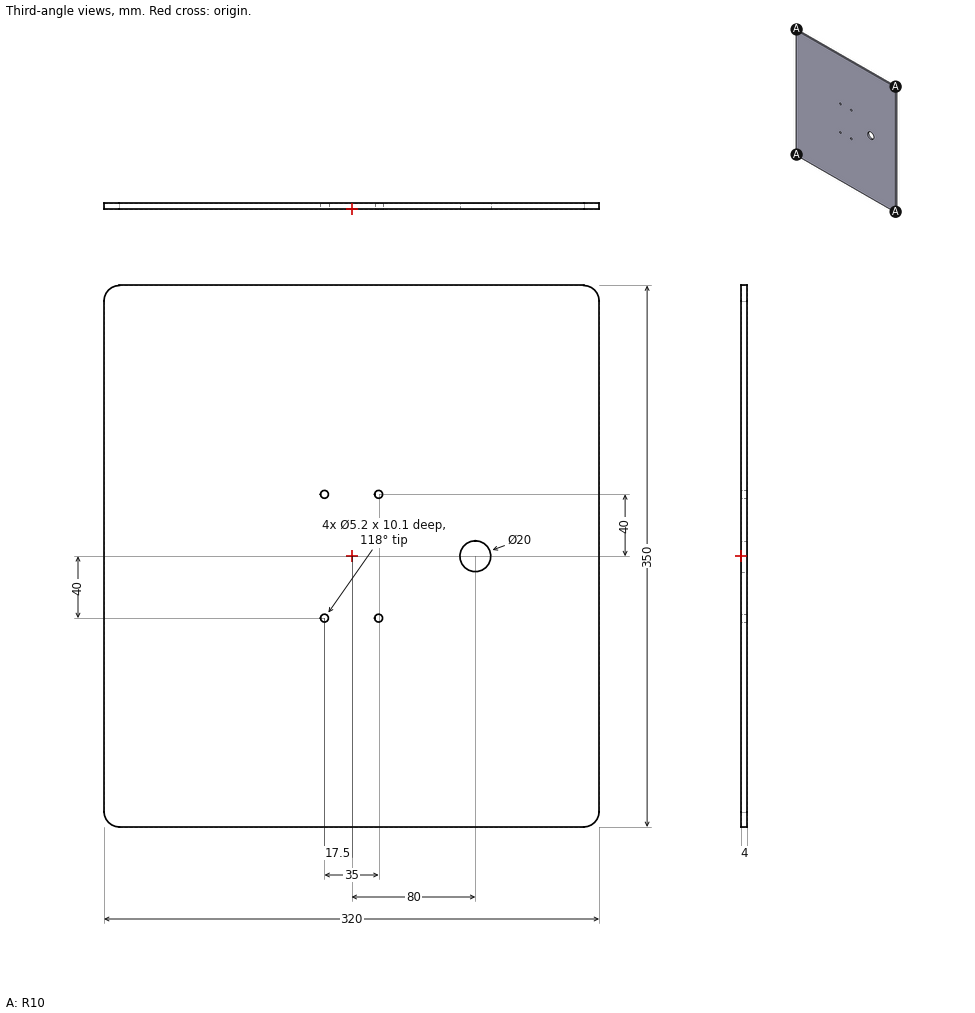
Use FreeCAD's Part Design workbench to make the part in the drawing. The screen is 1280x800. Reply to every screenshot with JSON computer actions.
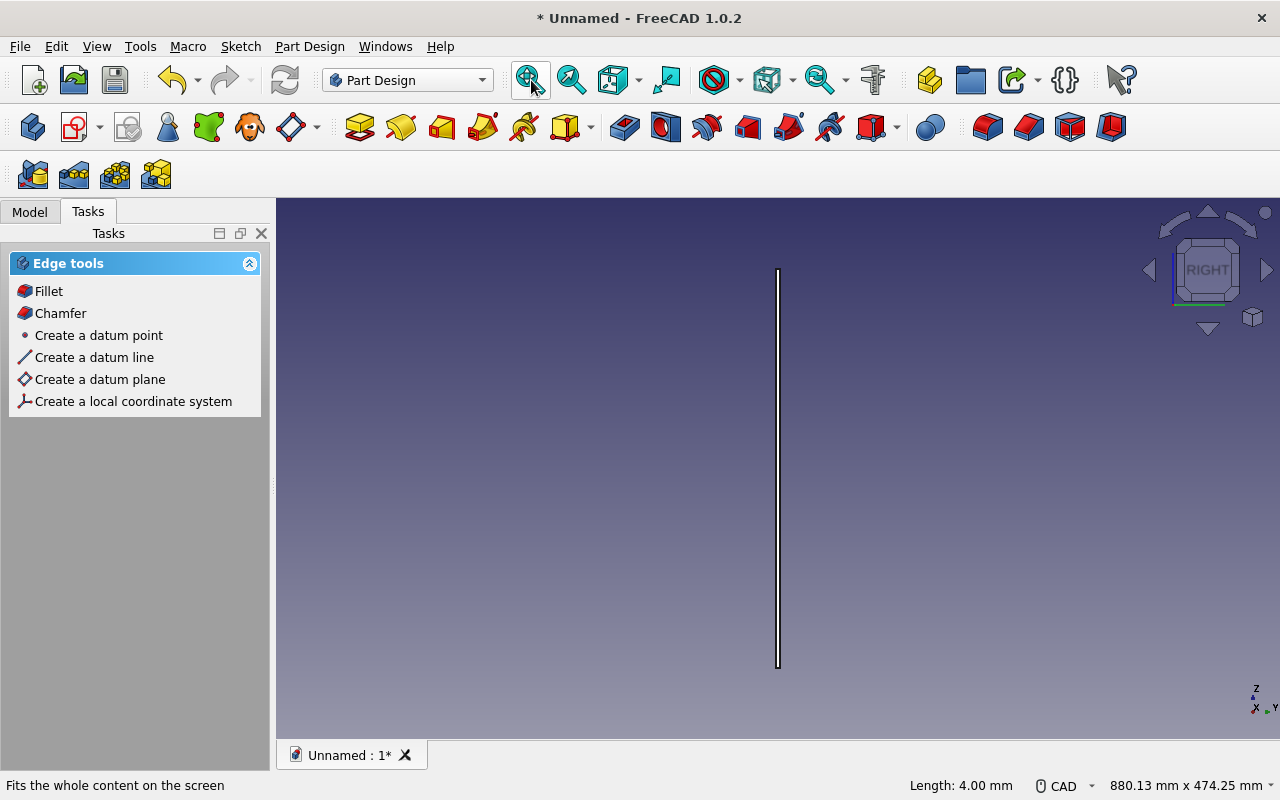
{"action": "scroll", "coordinate": [778, 667], "scroll_direction": "up", "scroll_amount": 11}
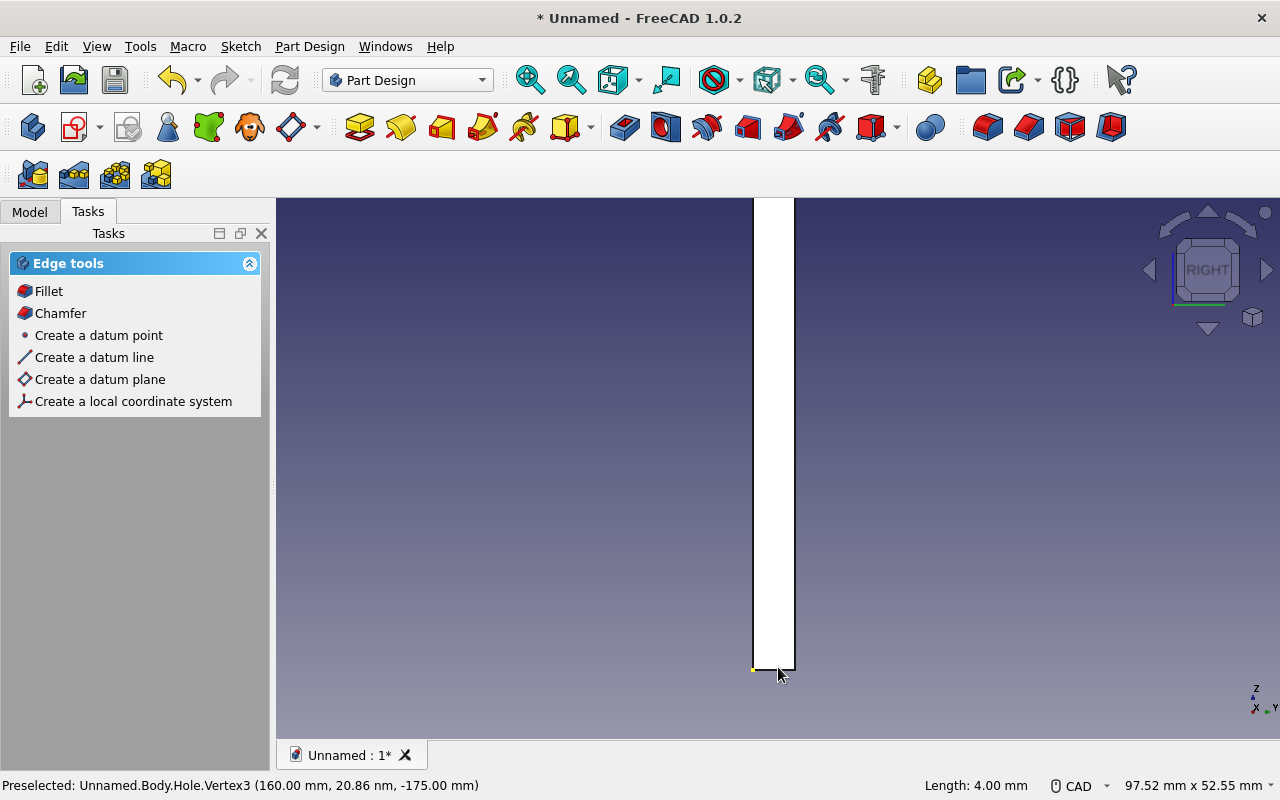
{"action": "left_click", "coordinate": [774, 669], "text": "ctrl"}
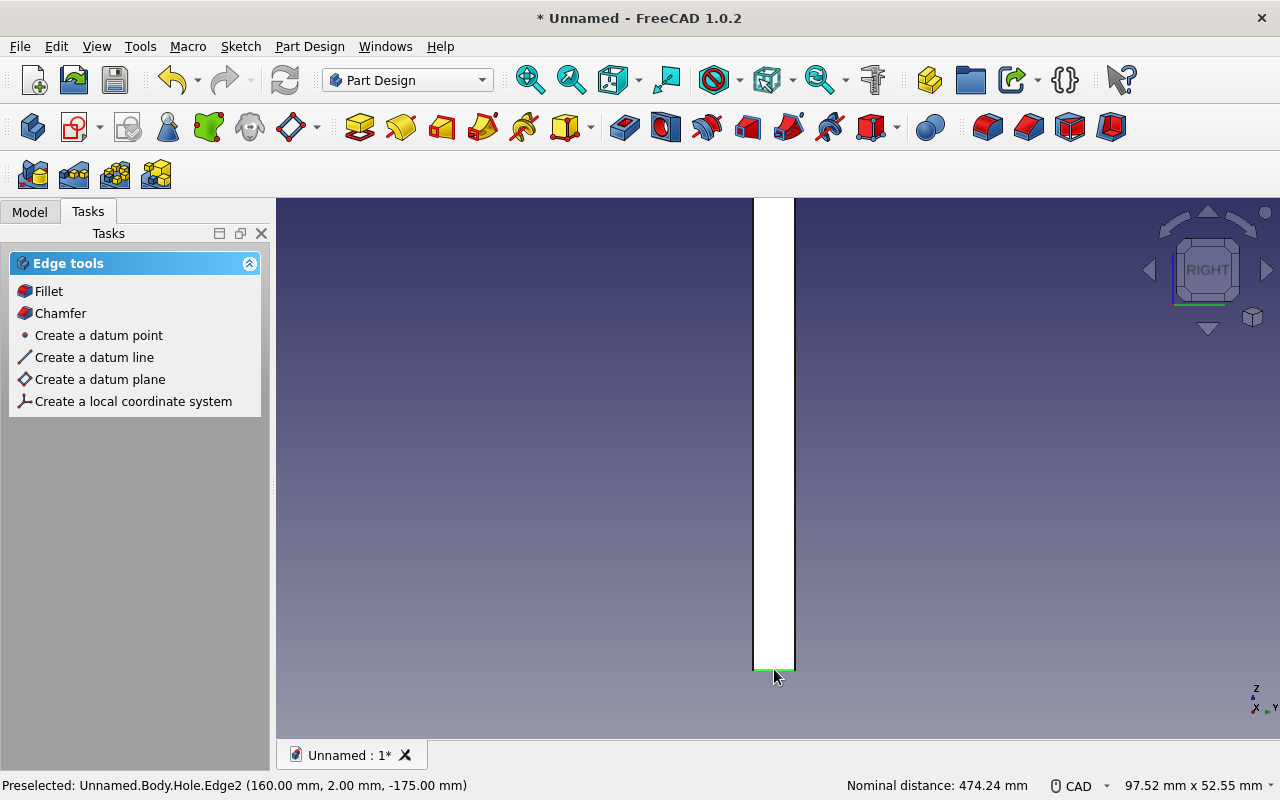
{"action": "left_click", "coordinate": [531, 80]}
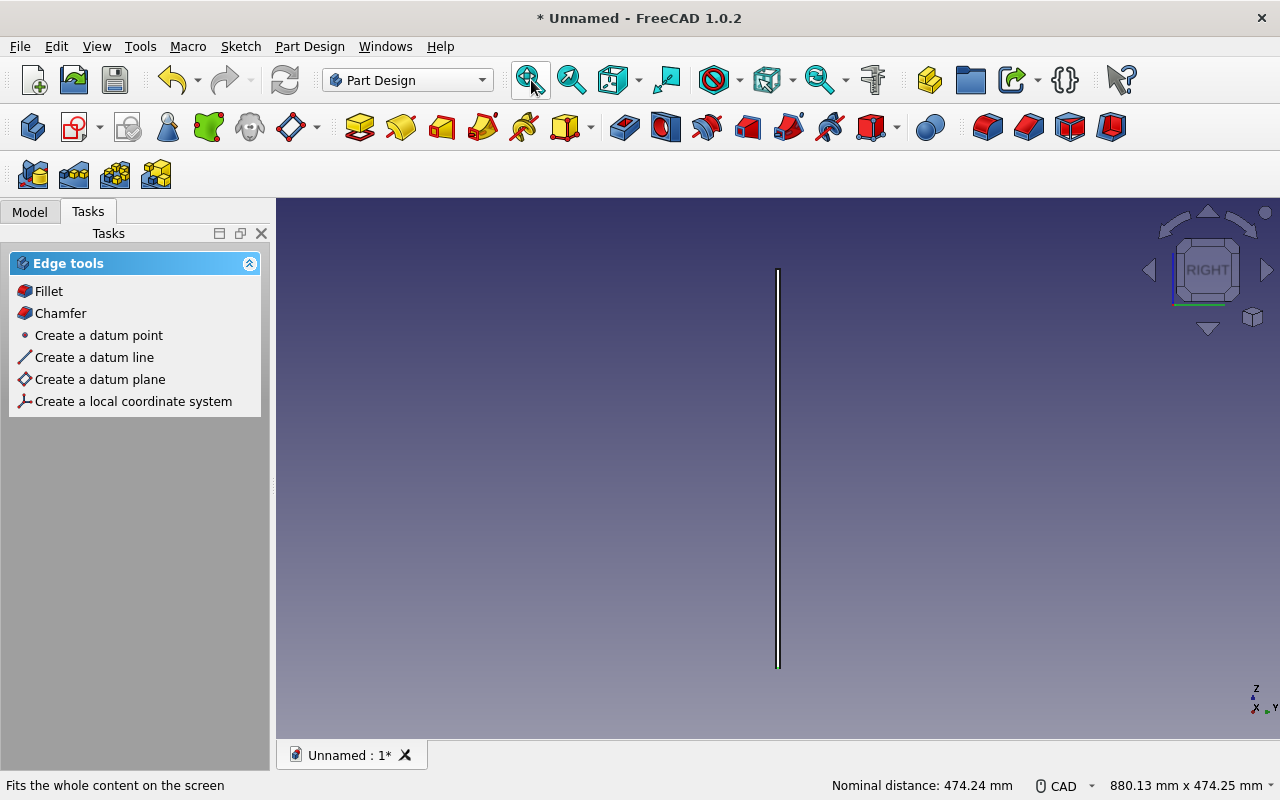
{"action": "key", "text": "5"}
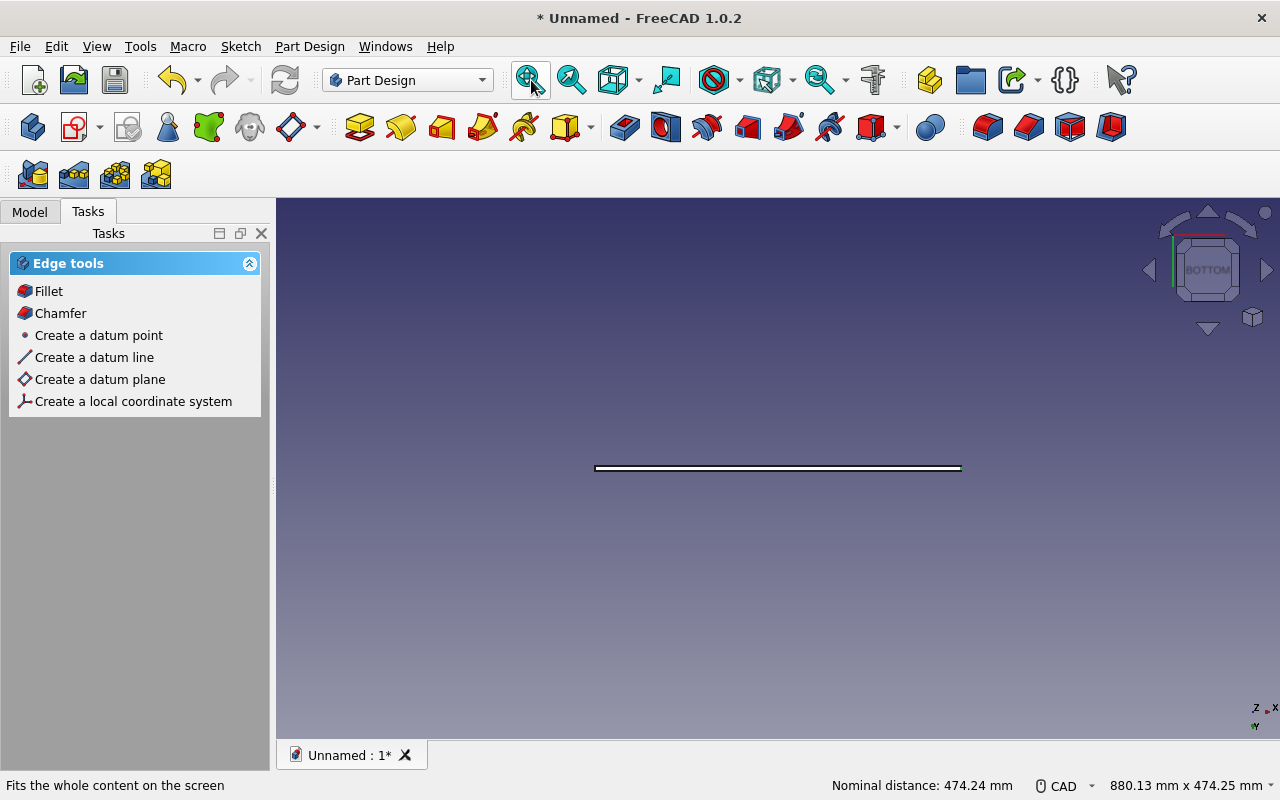
{"action": "left_click", "coordinate": [531, 80]}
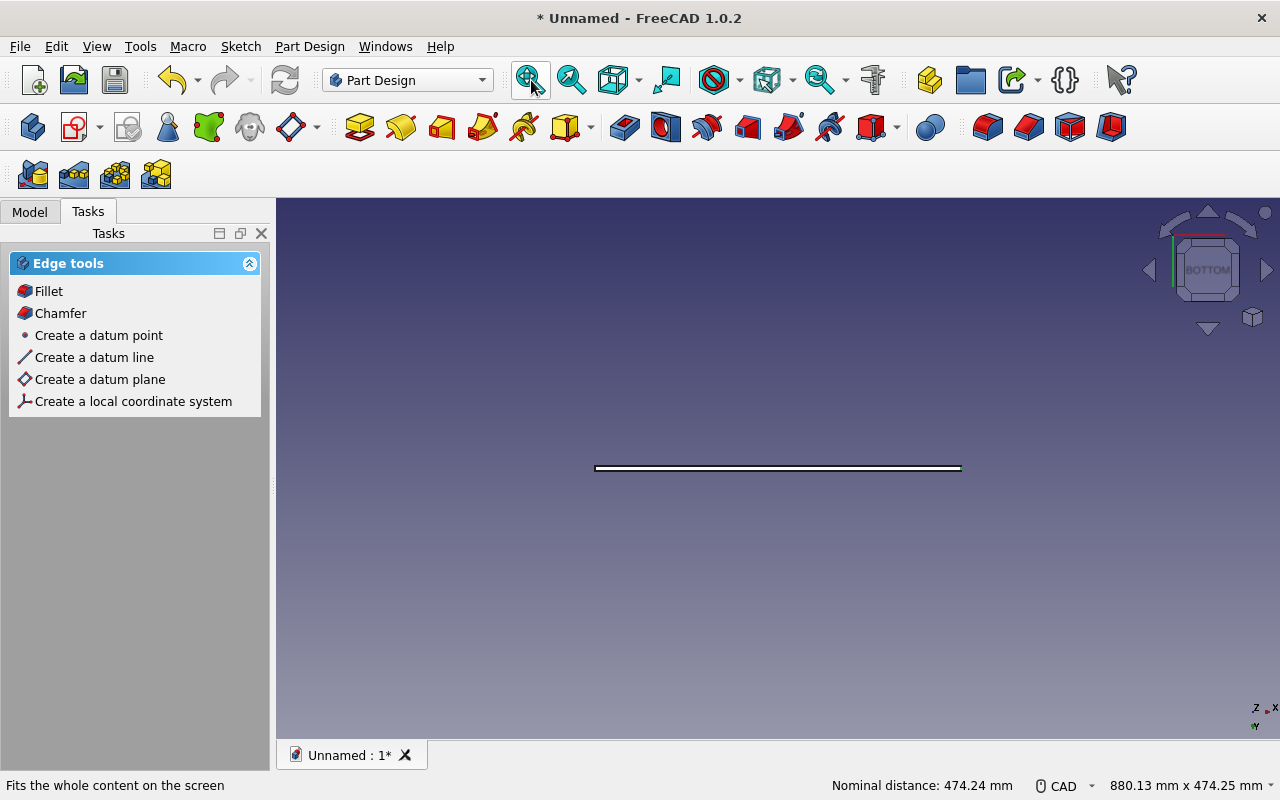
{"action": "scroll", "coordinate": [595, 467], "scroll_direction": "up", "scroll_amount": 11}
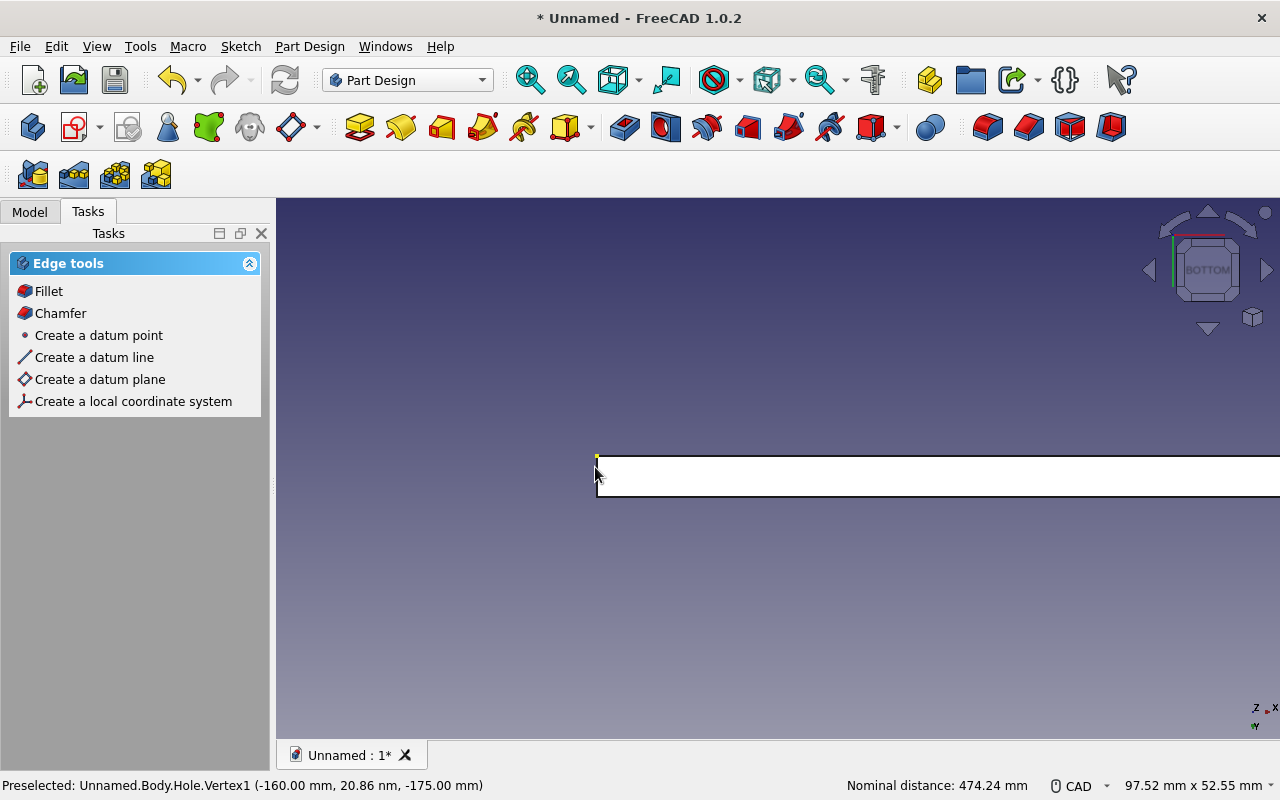
{"action": "left_click", "coordinate": [597, 476], "text": "ctrl"}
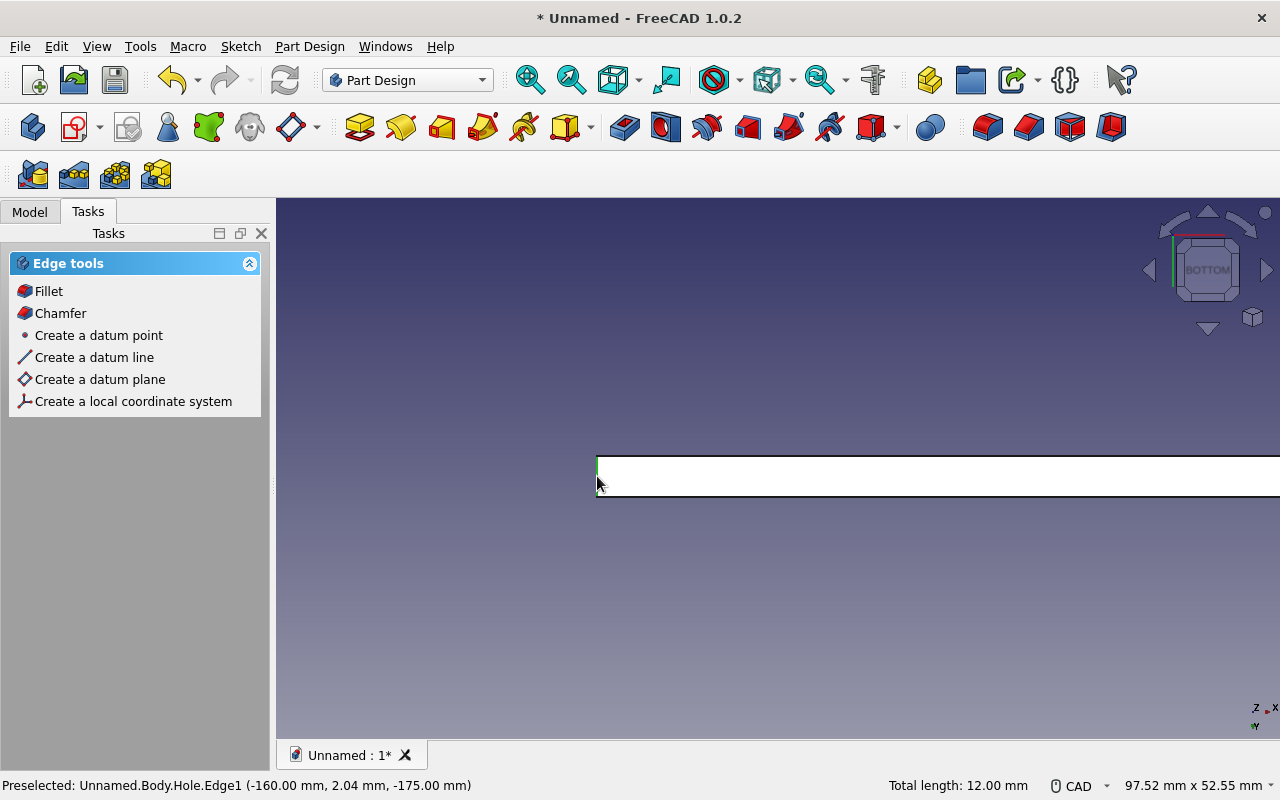
{"action": "left_click", "coordinate": [531, 80]}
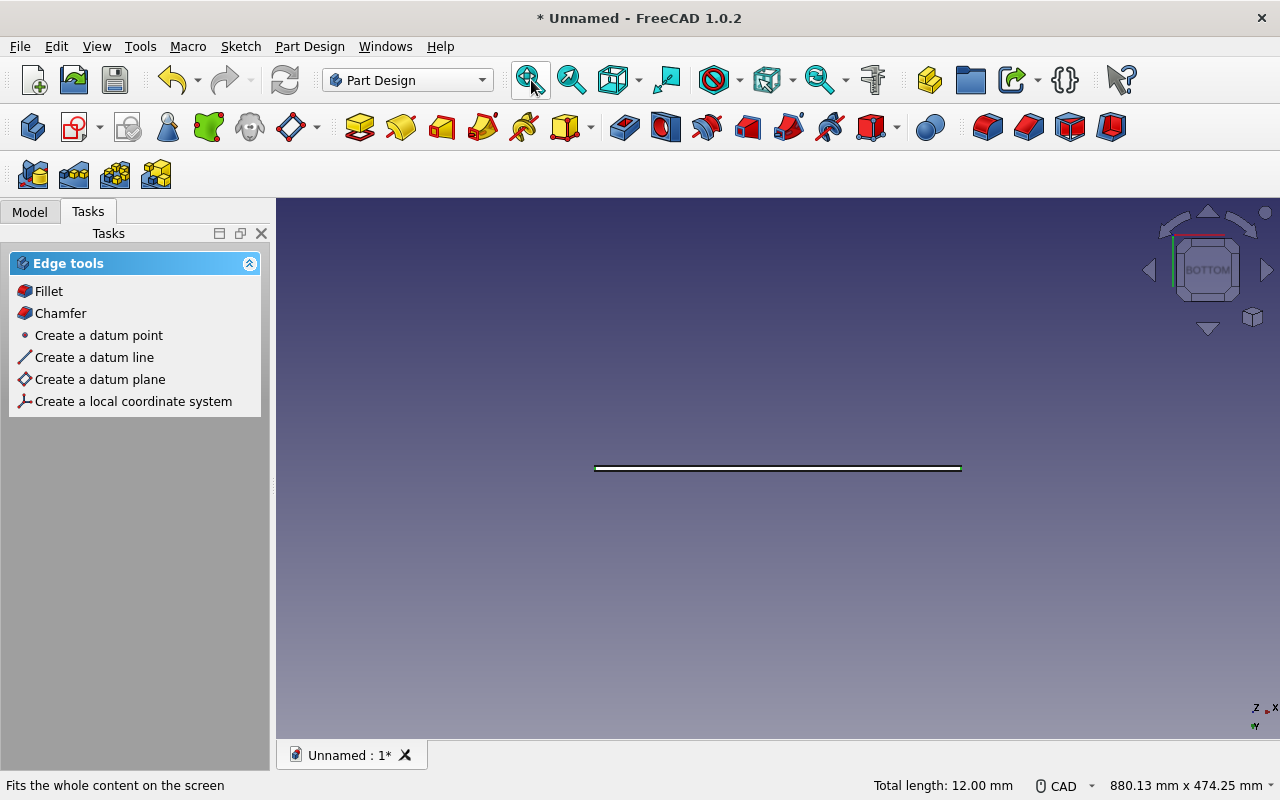
{"action": "key", "text": "4"}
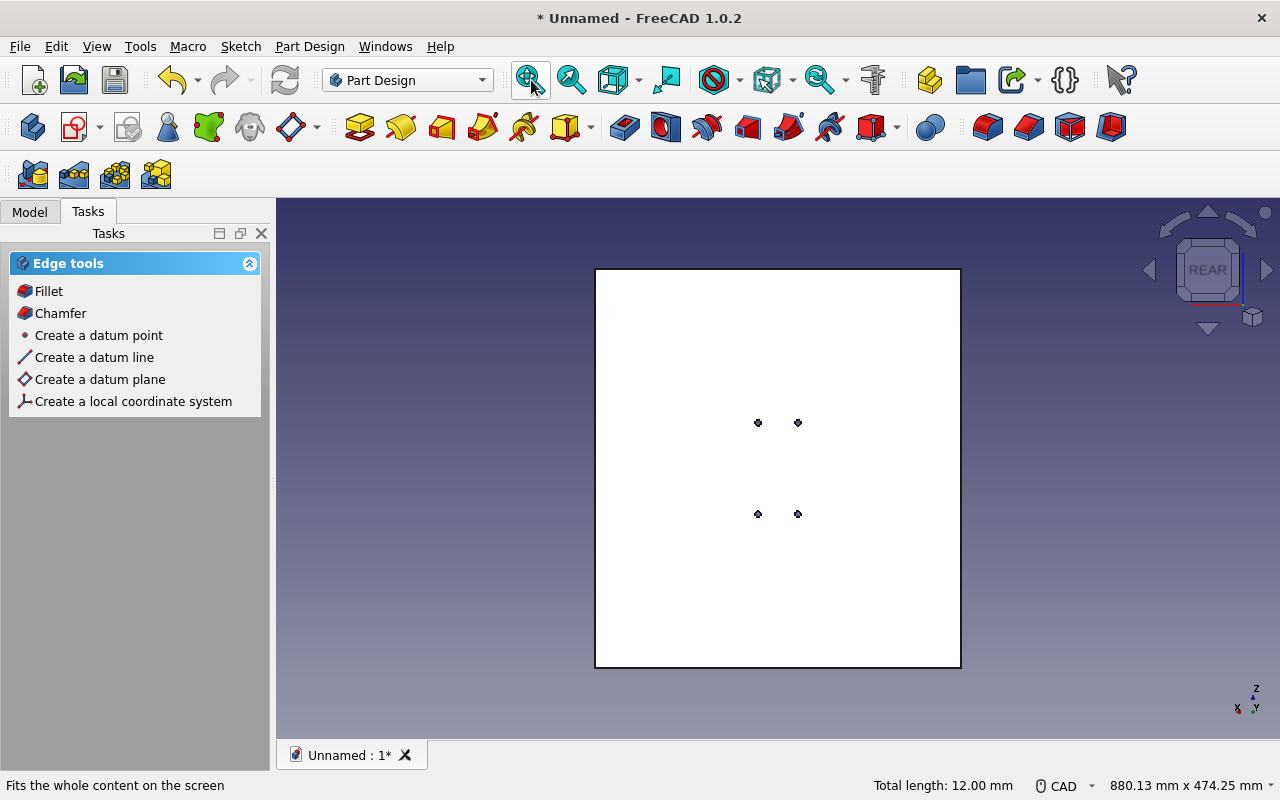
{"action": "scroll", "coordinate": [595, 268], "scroll_direction": "up", "scroll_amount": 11}